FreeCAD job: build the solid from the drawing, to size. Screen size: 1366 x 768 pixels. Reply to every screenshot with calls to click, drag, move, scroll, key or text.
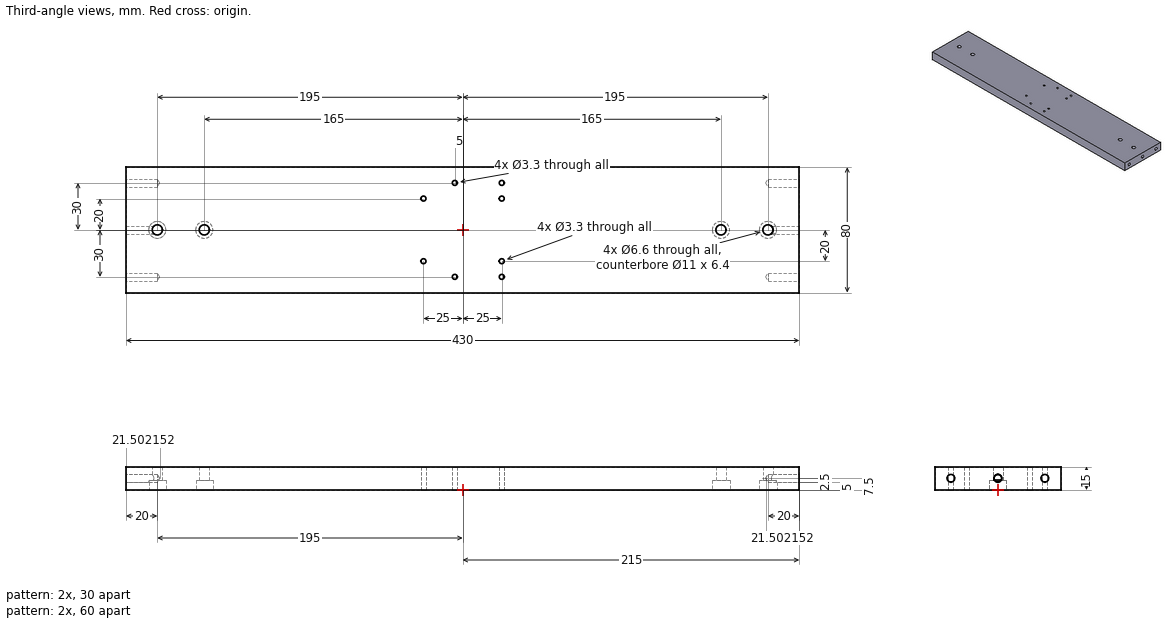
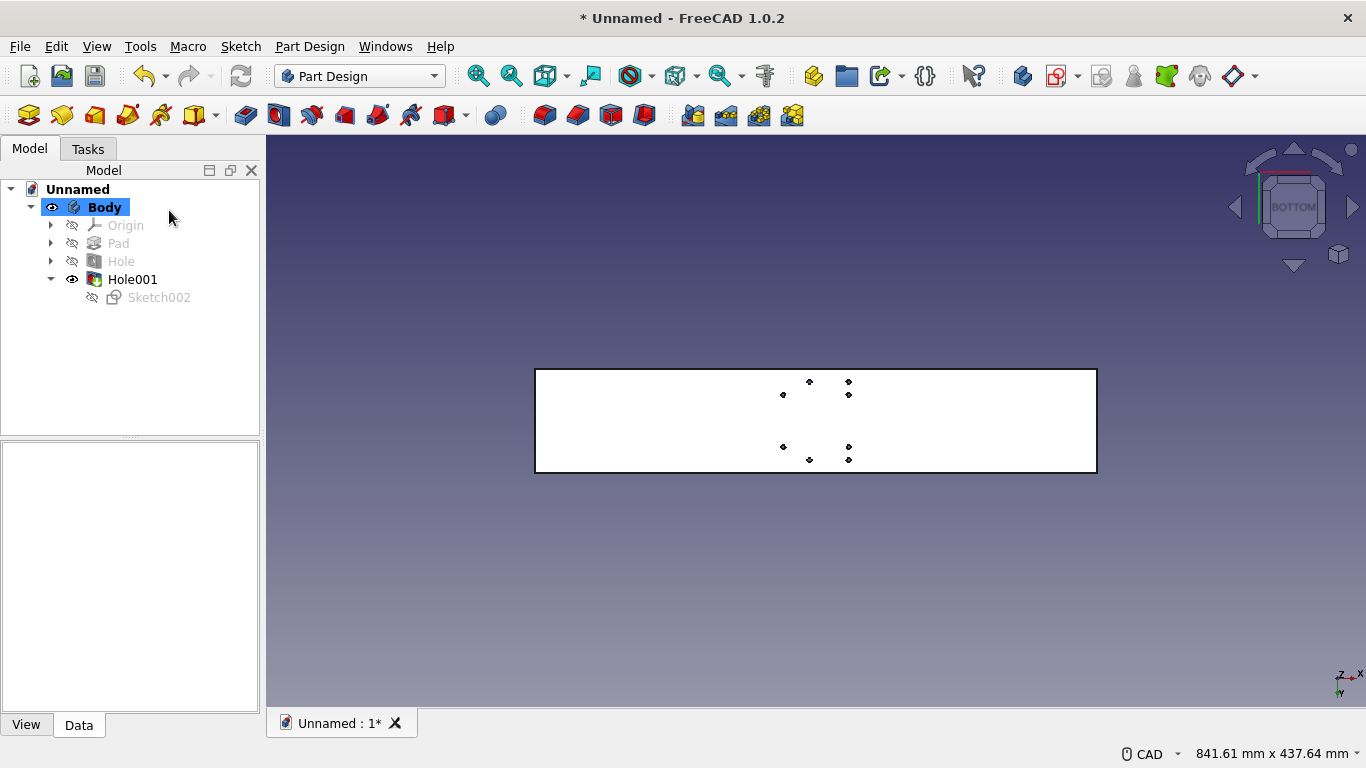
click(977, 420)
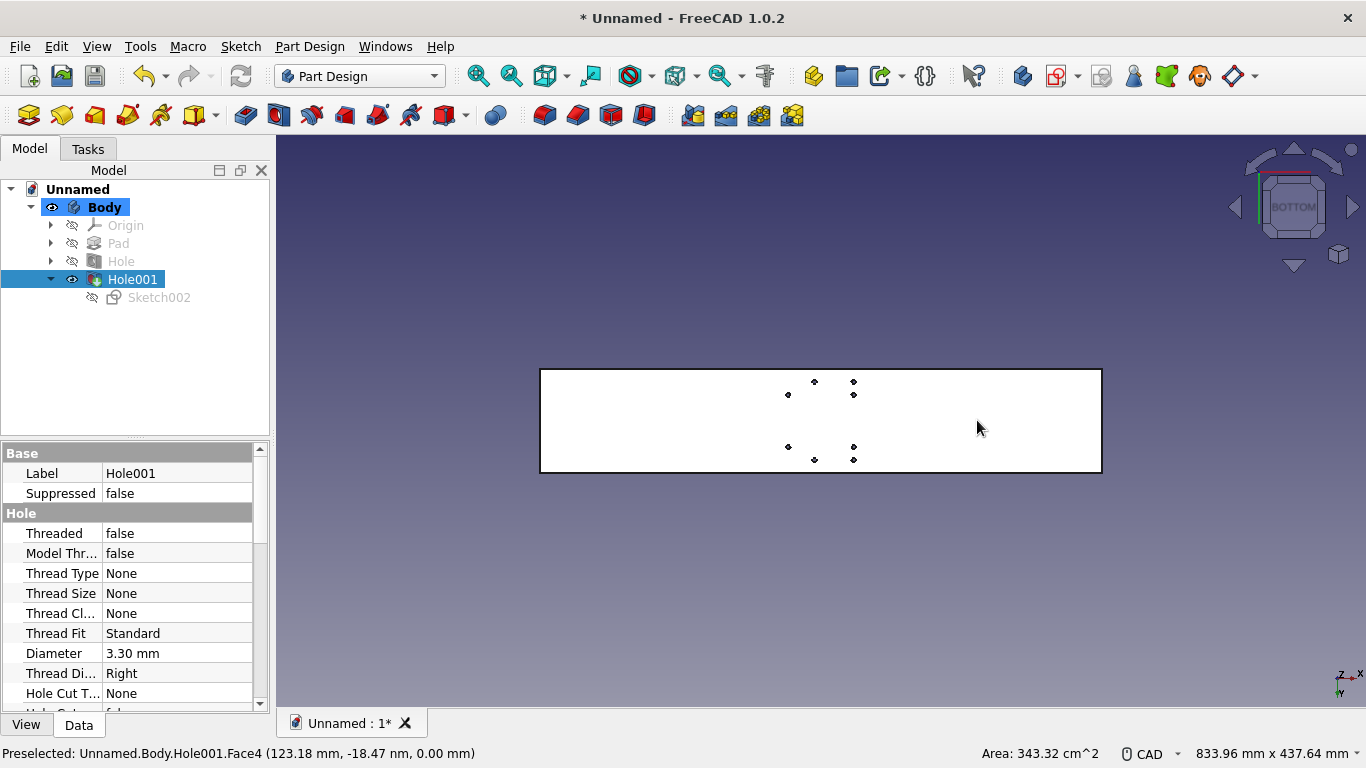
click(1056, 76)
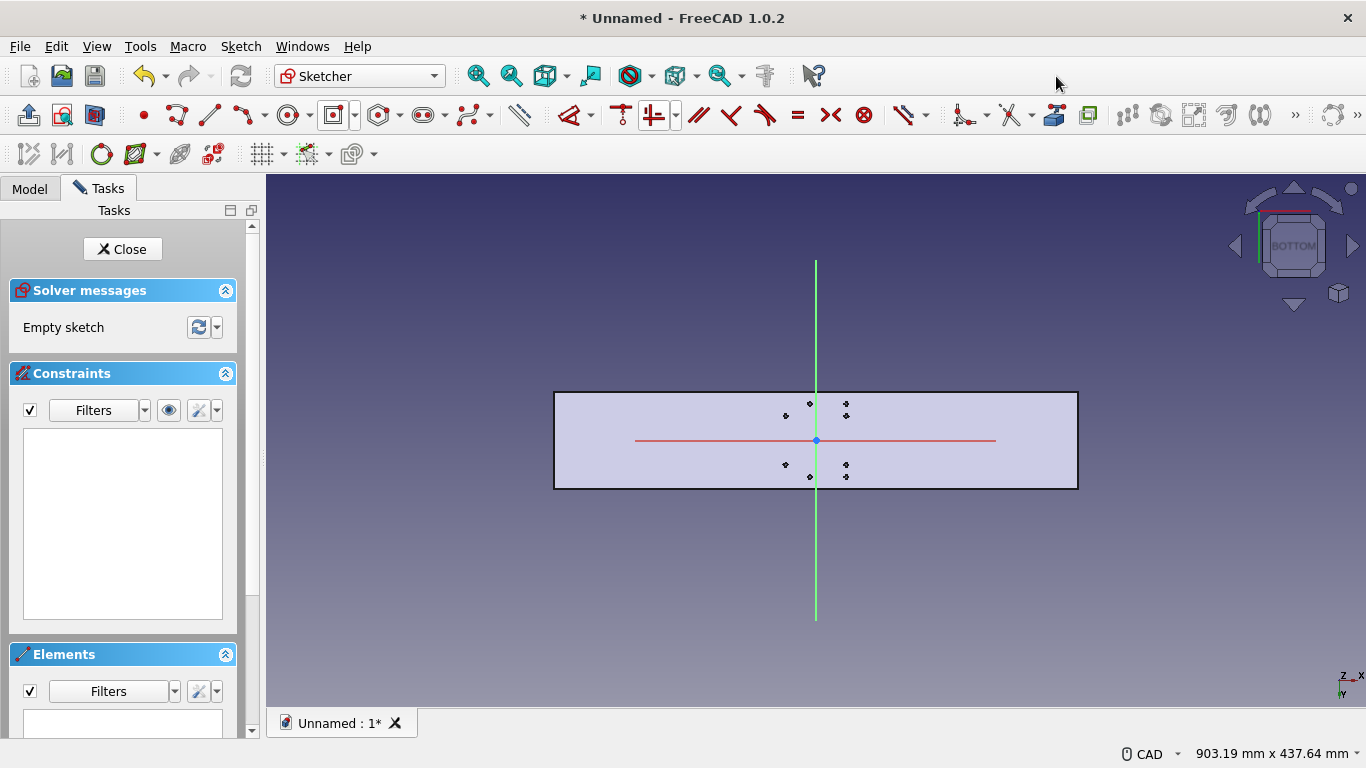
click(288, 116)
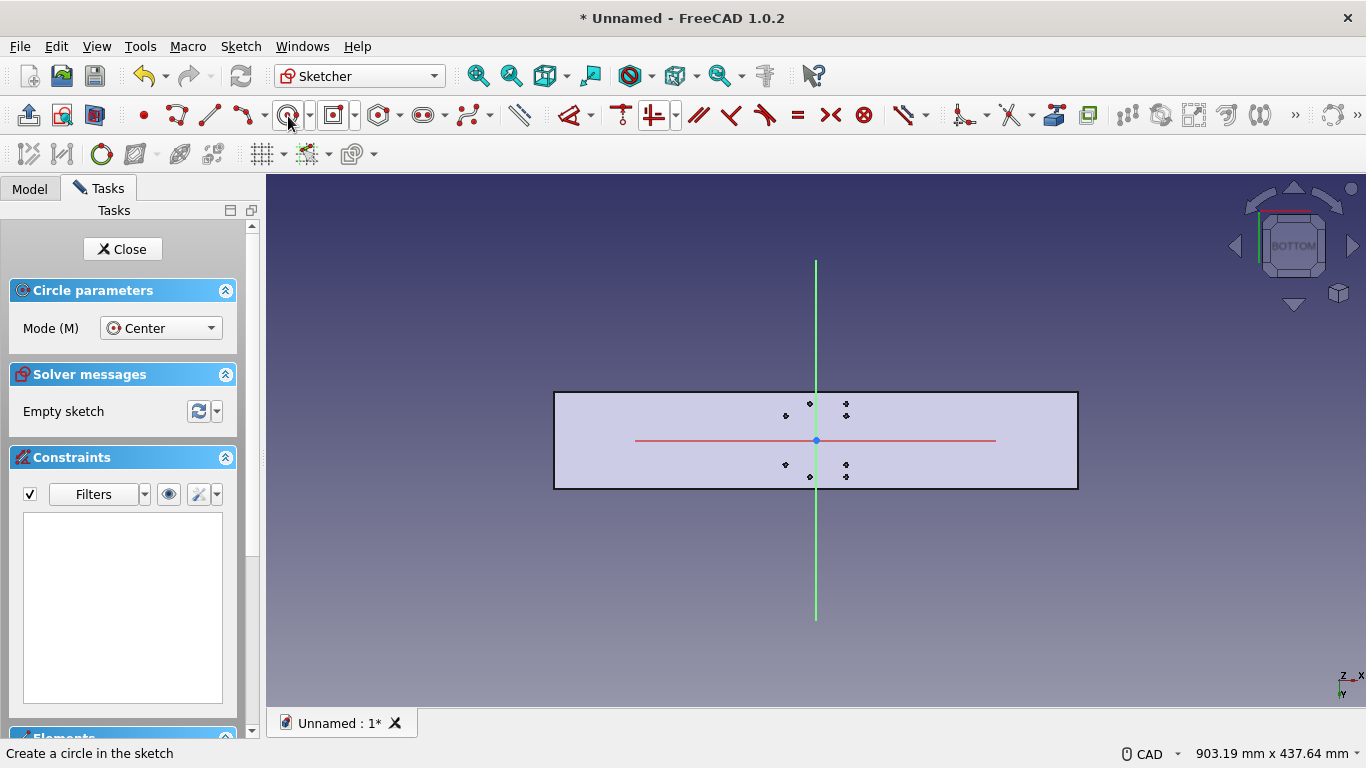
scroll(1053, 441, up, 9)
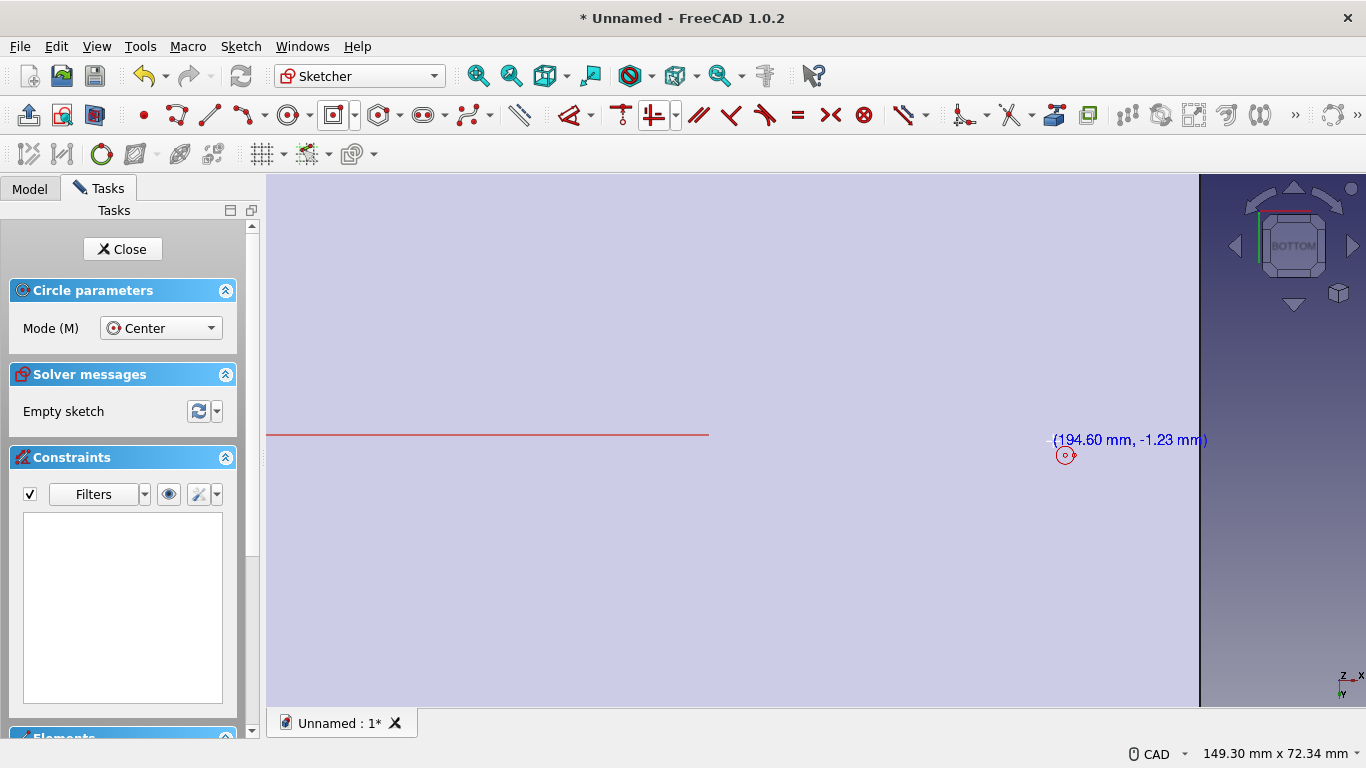
scroll(1034, 442, down, 8)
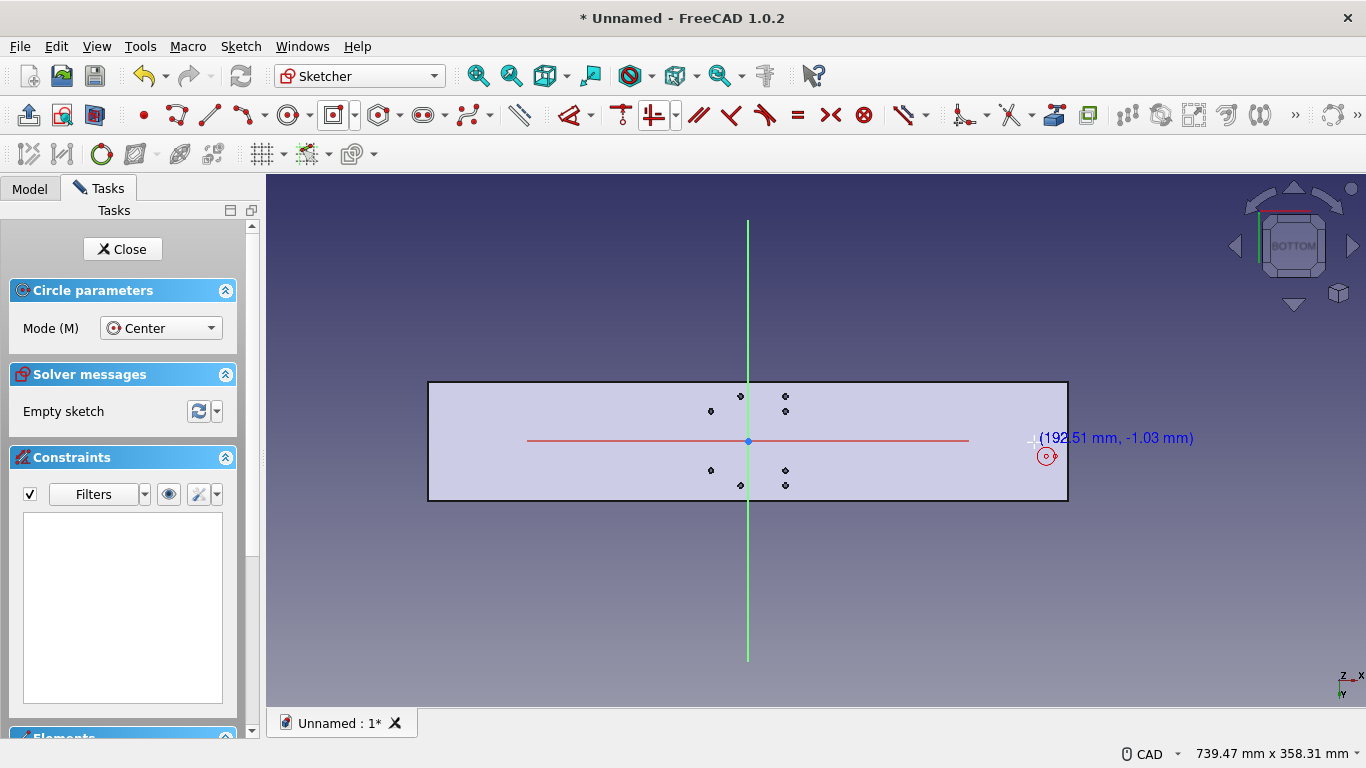
click(1038, 441)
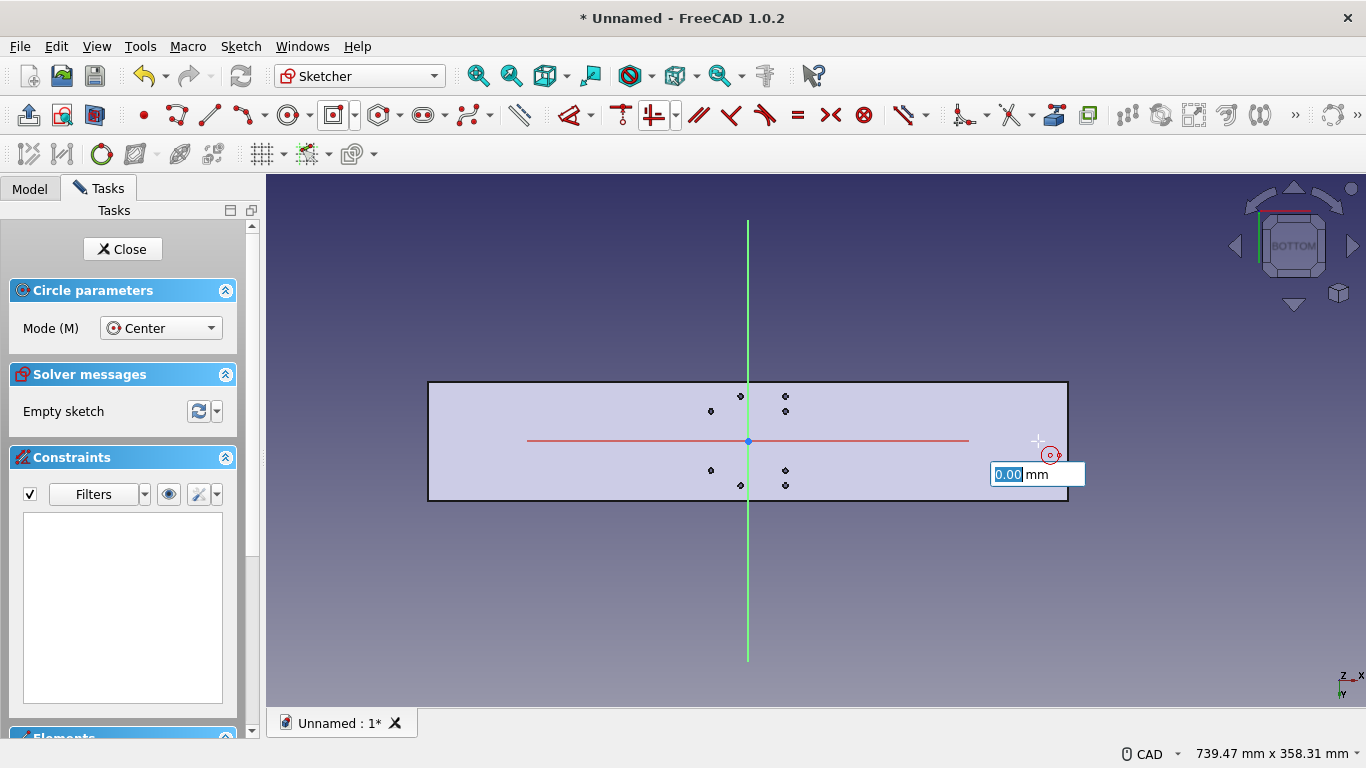
scroll(1037, 446, up, 7)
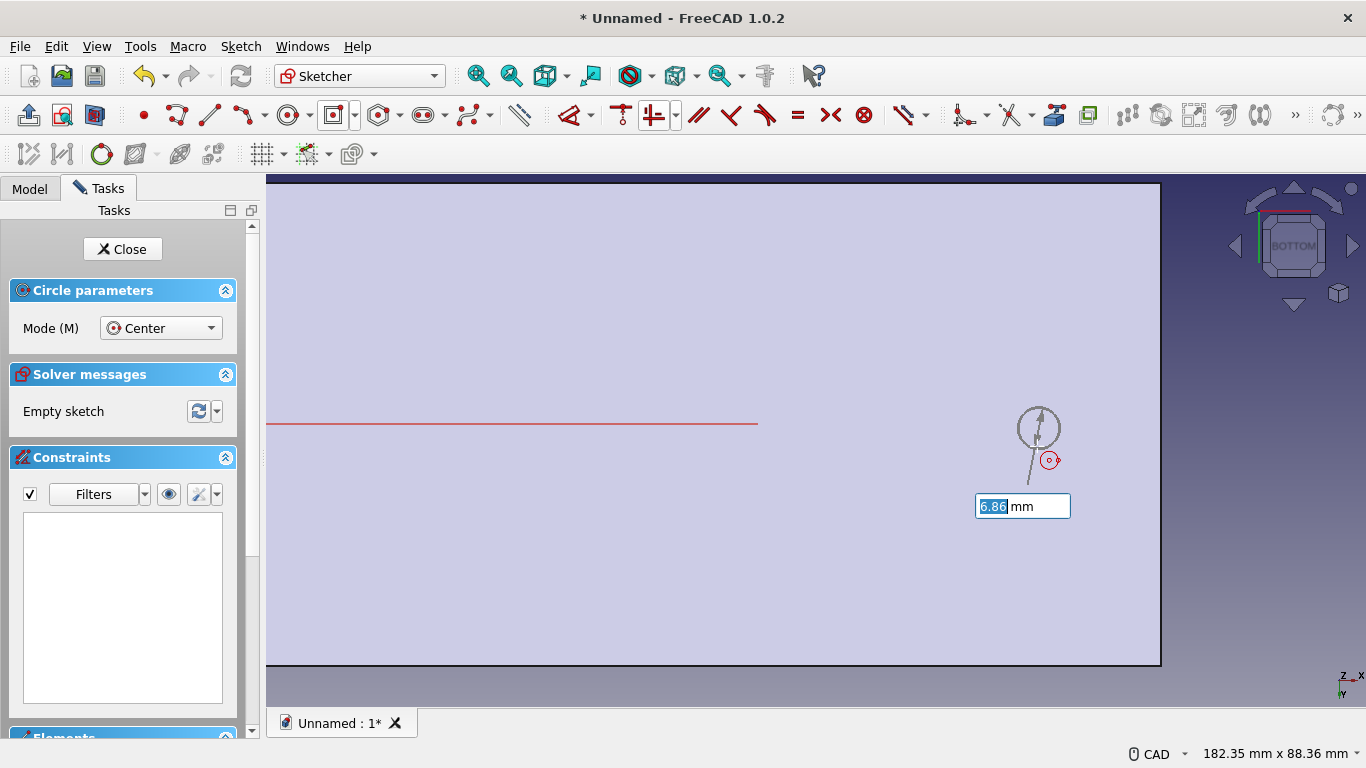
click(1033, 443)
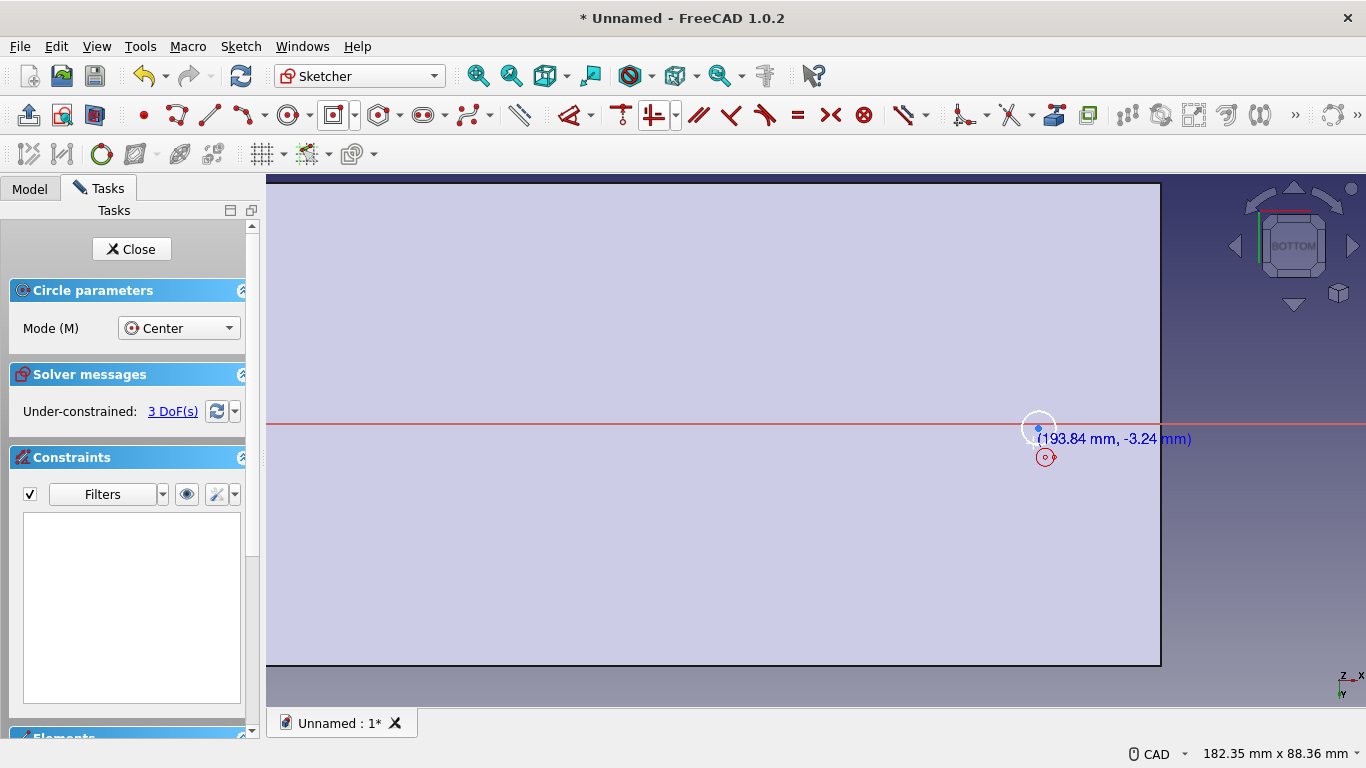
scroll(1037, 446, down, 7)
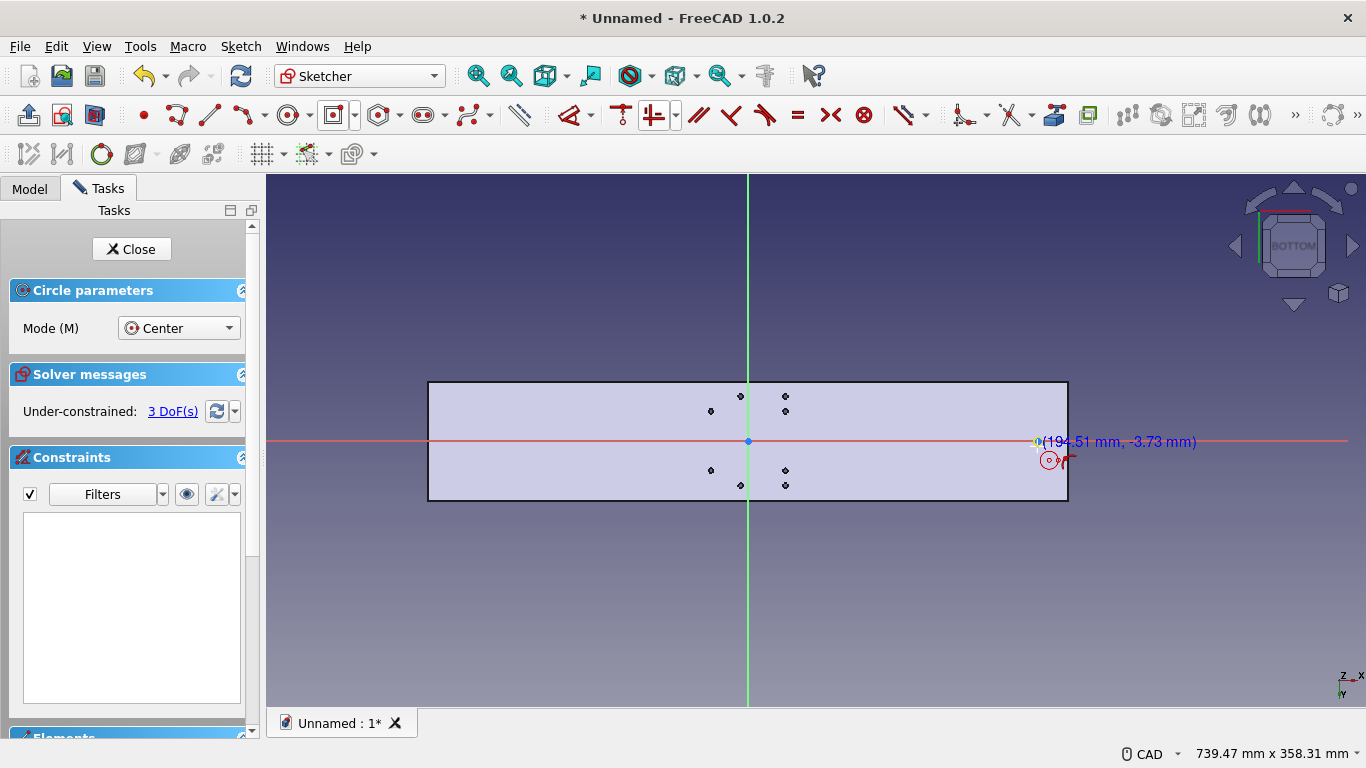
click(994, 441)